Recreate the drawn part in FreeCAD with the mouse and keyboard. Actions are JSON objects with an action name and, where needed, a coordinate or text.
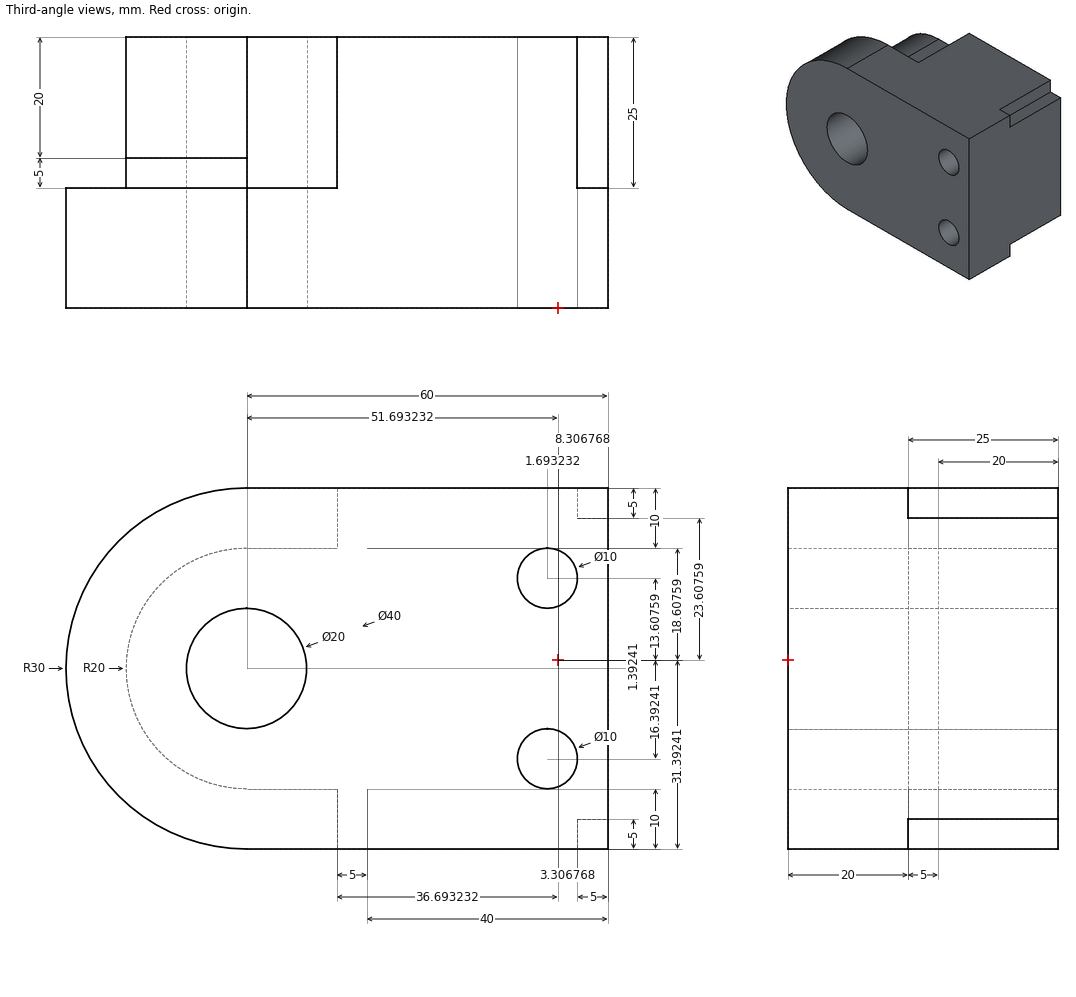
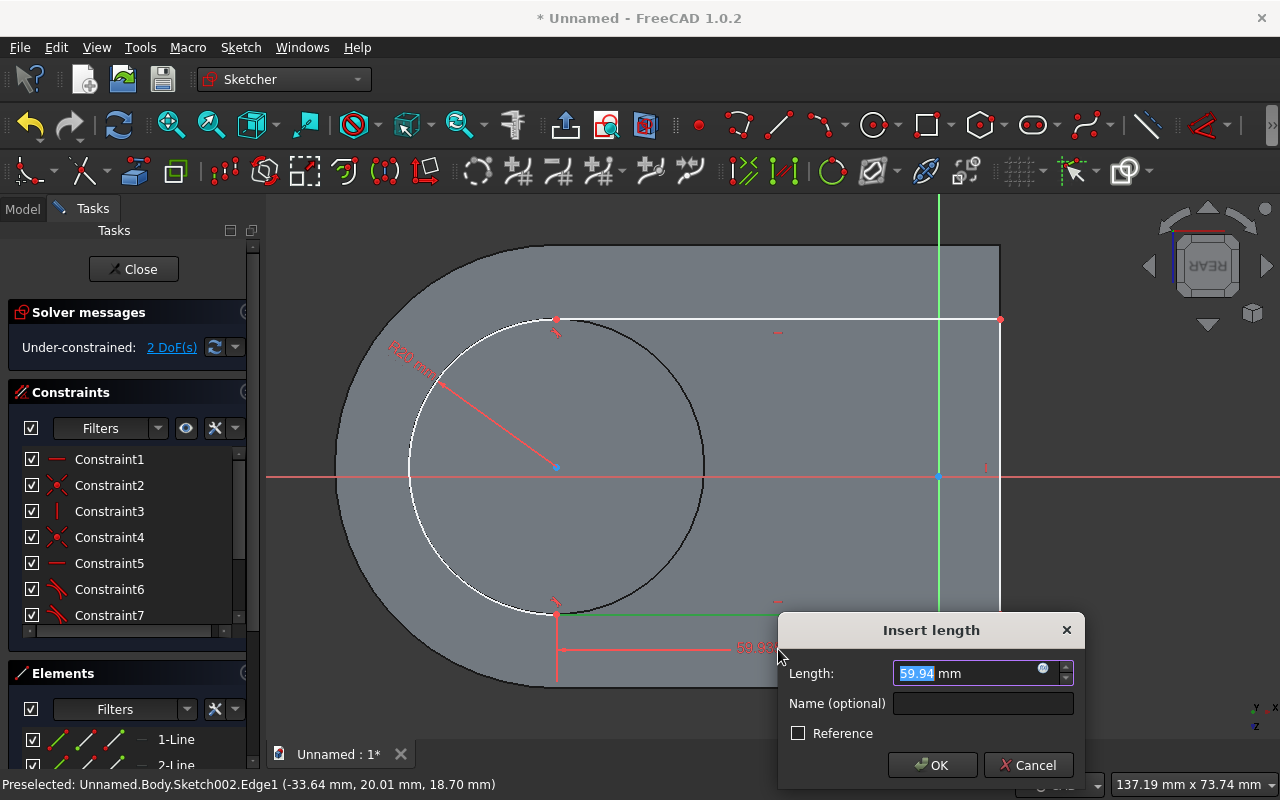
{"action": "type", "text": "60"}
{"action": "key", "text": "Return"}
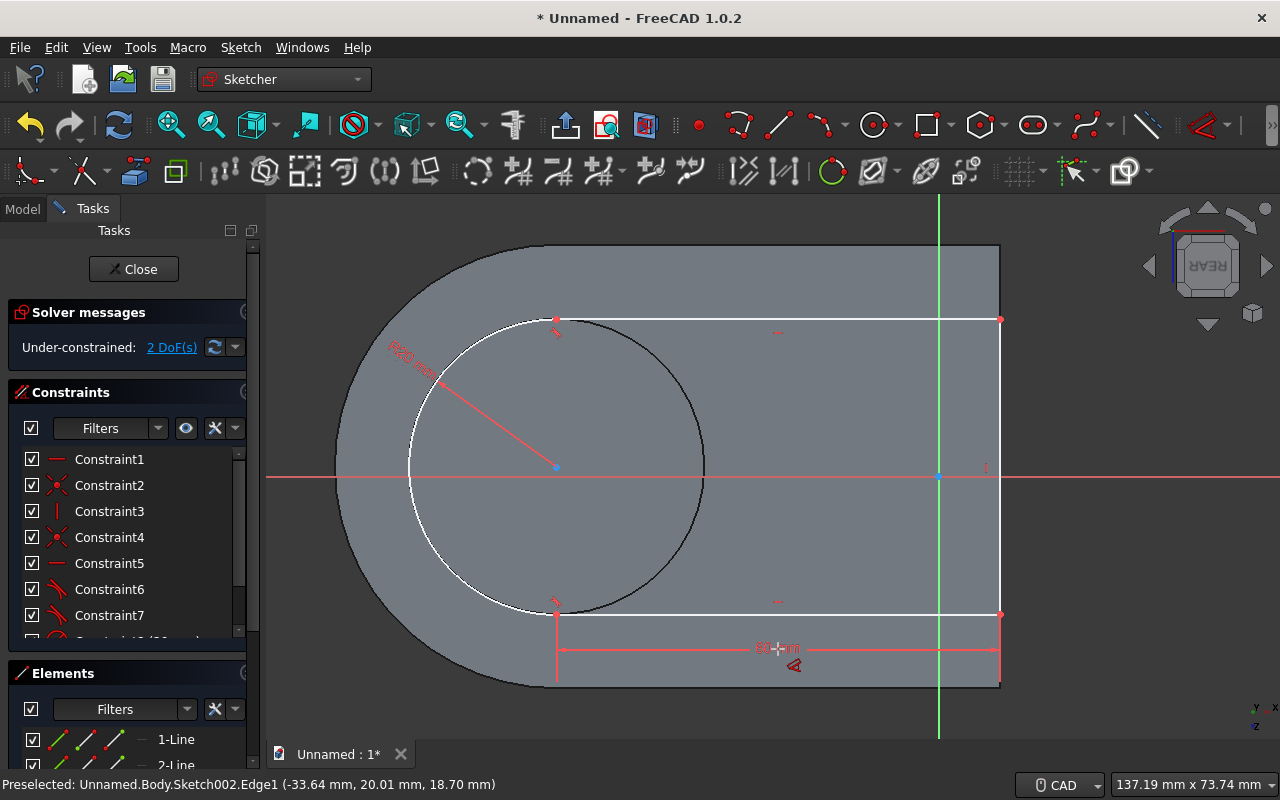
{"action": "scroll", "coordinate": [557, 467], "scroll_direction": "up", "scroll_amount": 7}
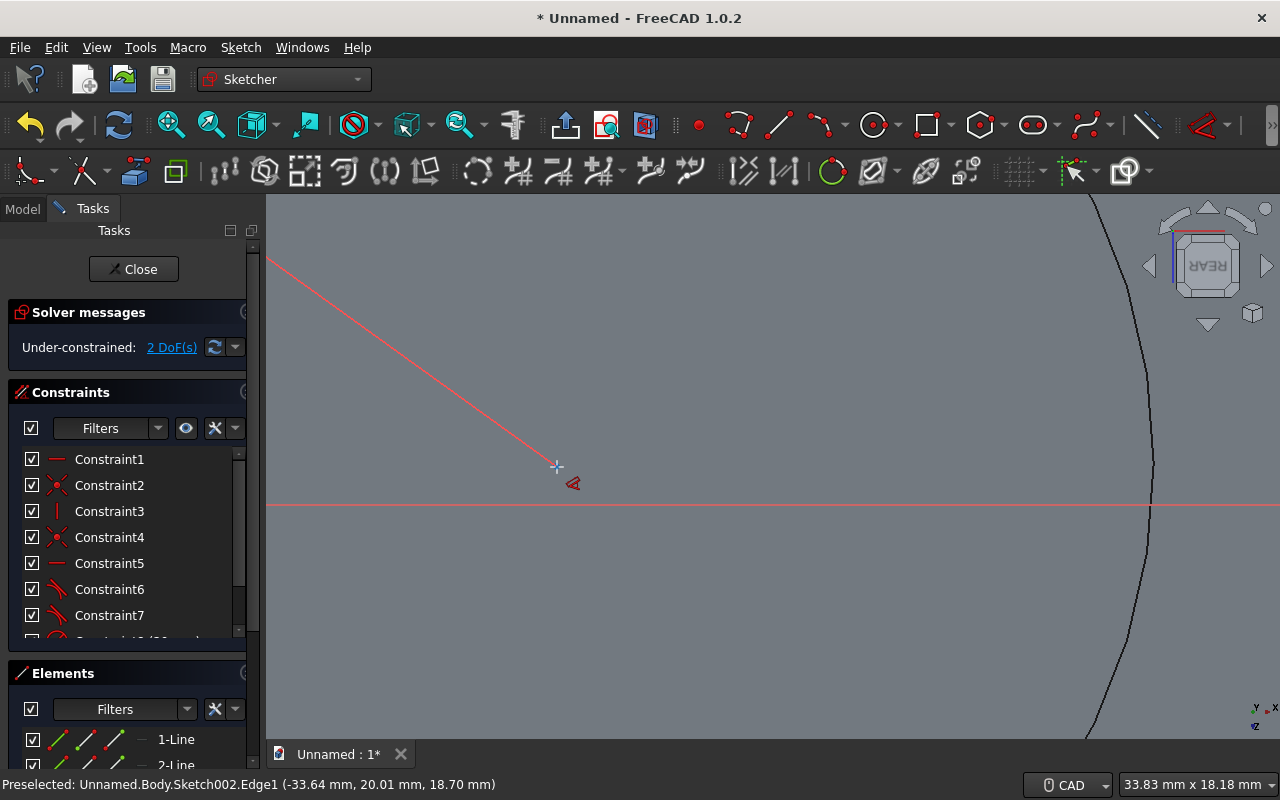
{"action": "left_click", "coordinate": [556, 466]}
{"action": "left_click", "coordinate": [522, 486]}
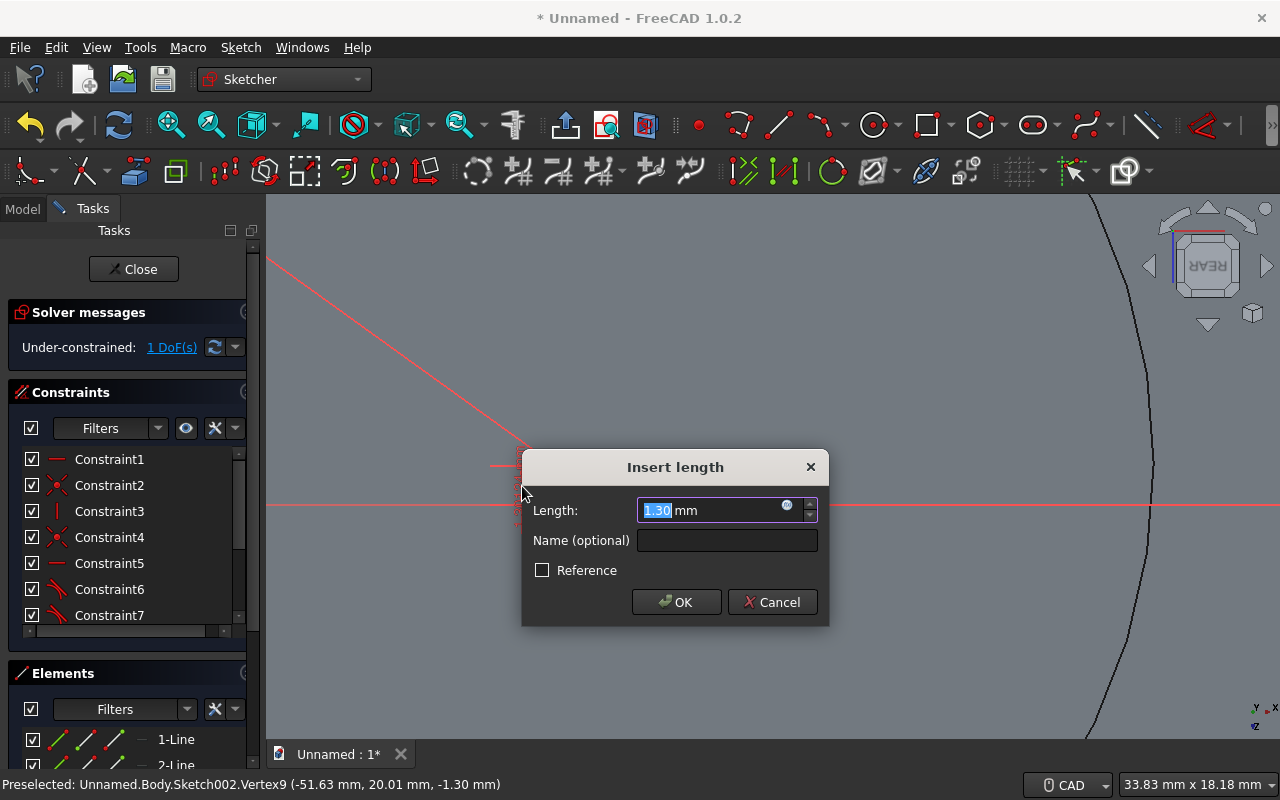
{"action": "type", "text": "1.39241"}
{"action": "key", "text": "Return"}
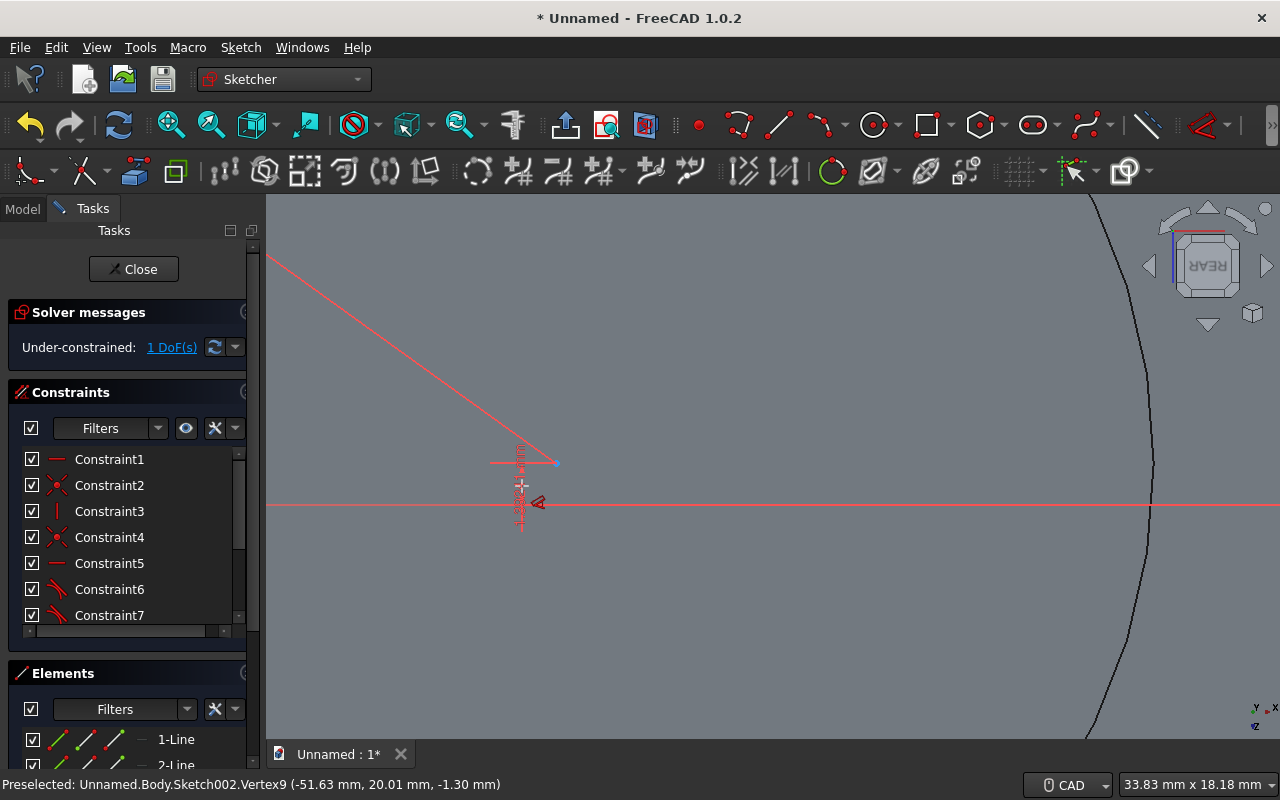
{"action": "scroll", "coordinate": [557, 468], "scroll_direction": "down", "scroll_amount": 7}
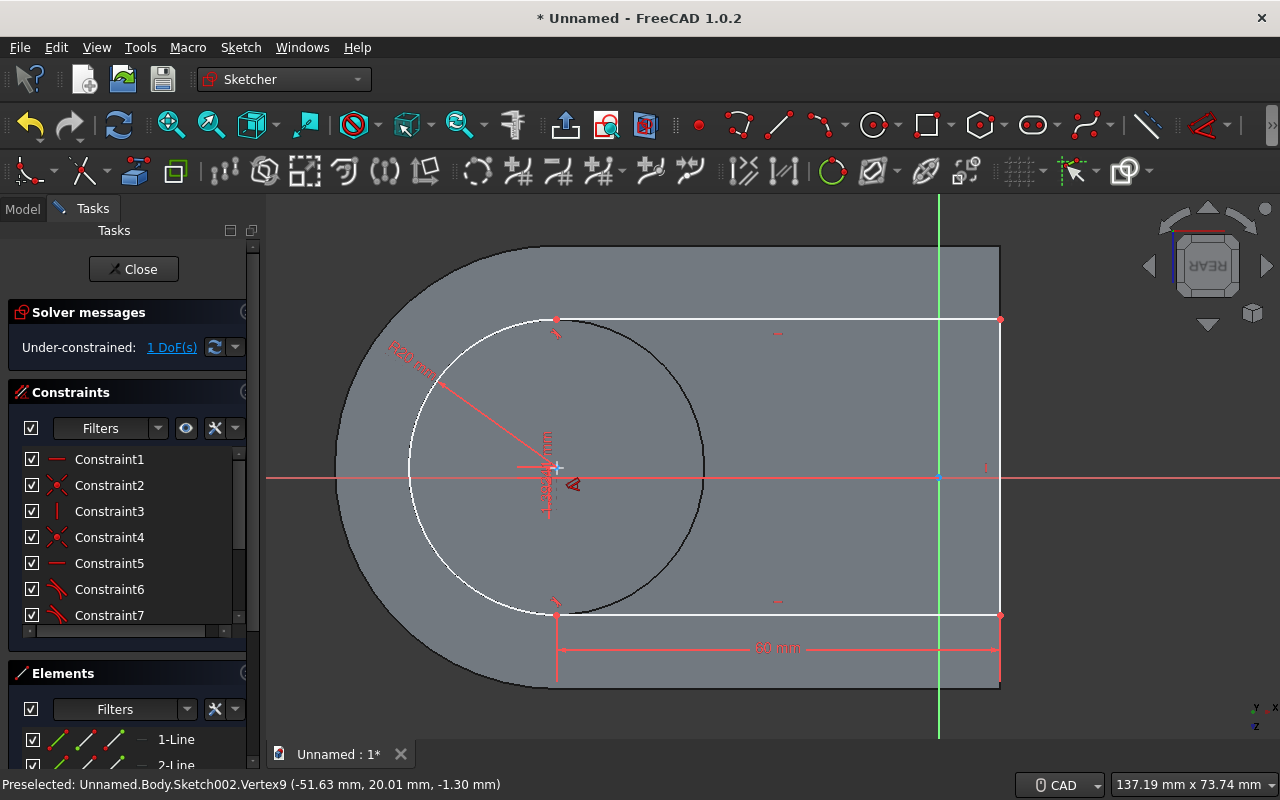
{"action": "left_click", "coordinate": [1000, 615]}
{"action": "left_click", "coordinate": [970, 649]}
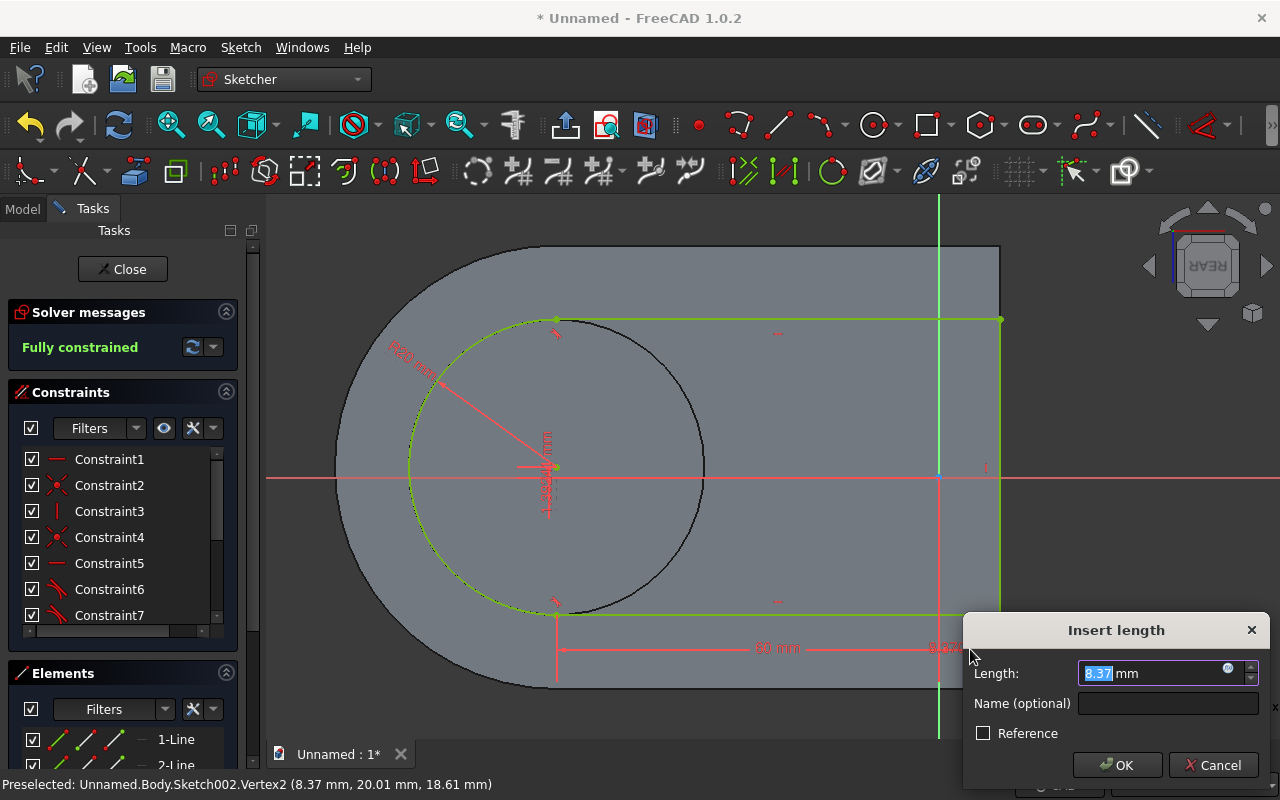
{"action": "type", "text": "8.306768"}
{"action": "key", "text": "Return"}
{"action": "key", "text": "Escape"}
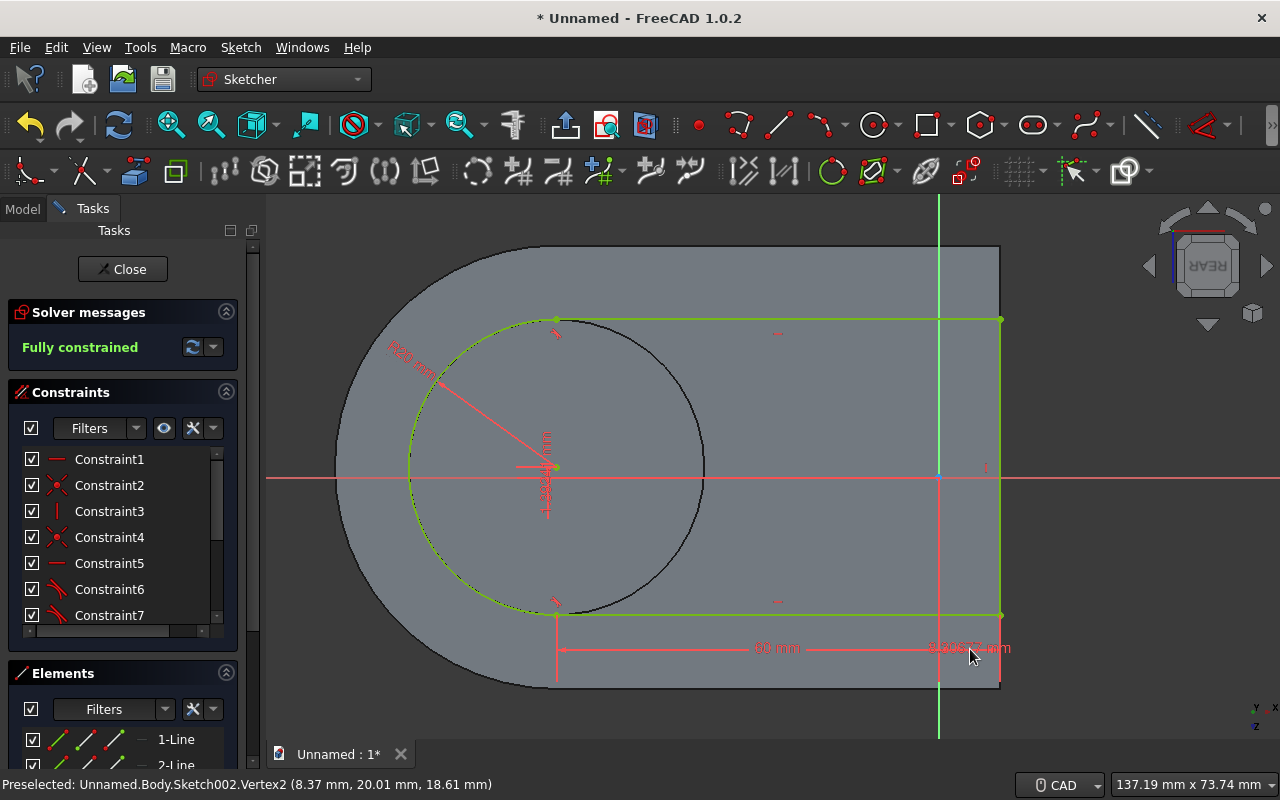
{"action": "left_click", "coordinate": [123, 269]}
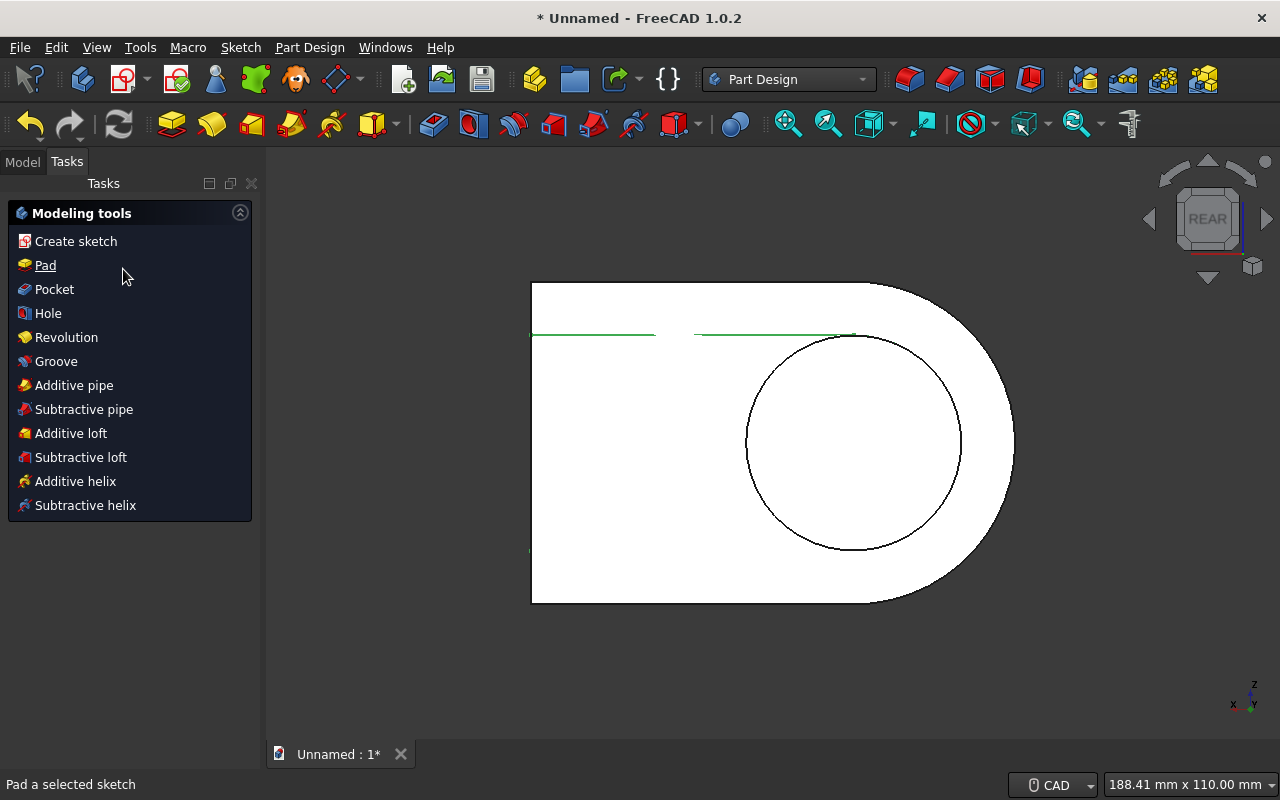
{"action": "left_click", "coordinate": [172, 124]}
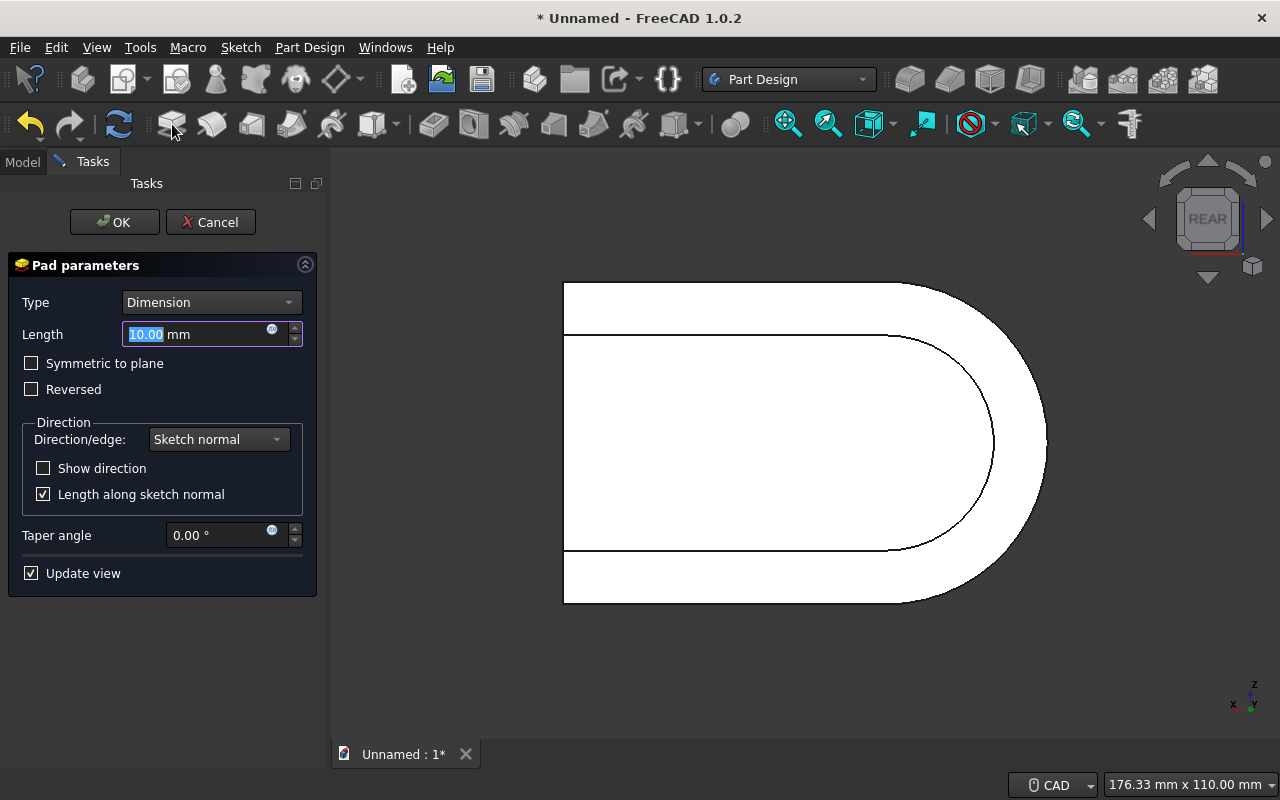
{"action": "type", "text": "5"}
{"action": "key", "text": "Tab"}